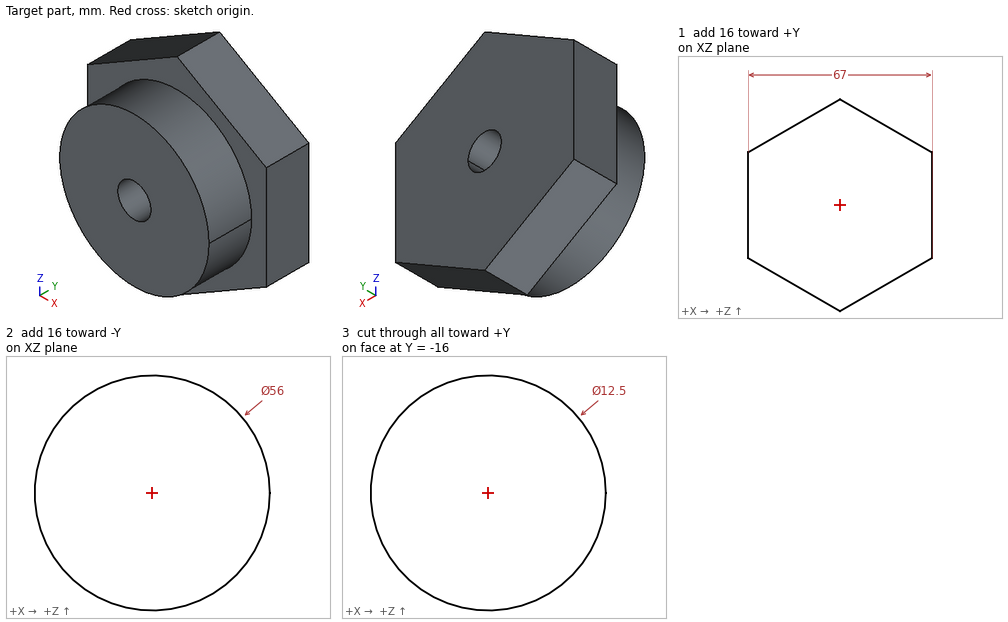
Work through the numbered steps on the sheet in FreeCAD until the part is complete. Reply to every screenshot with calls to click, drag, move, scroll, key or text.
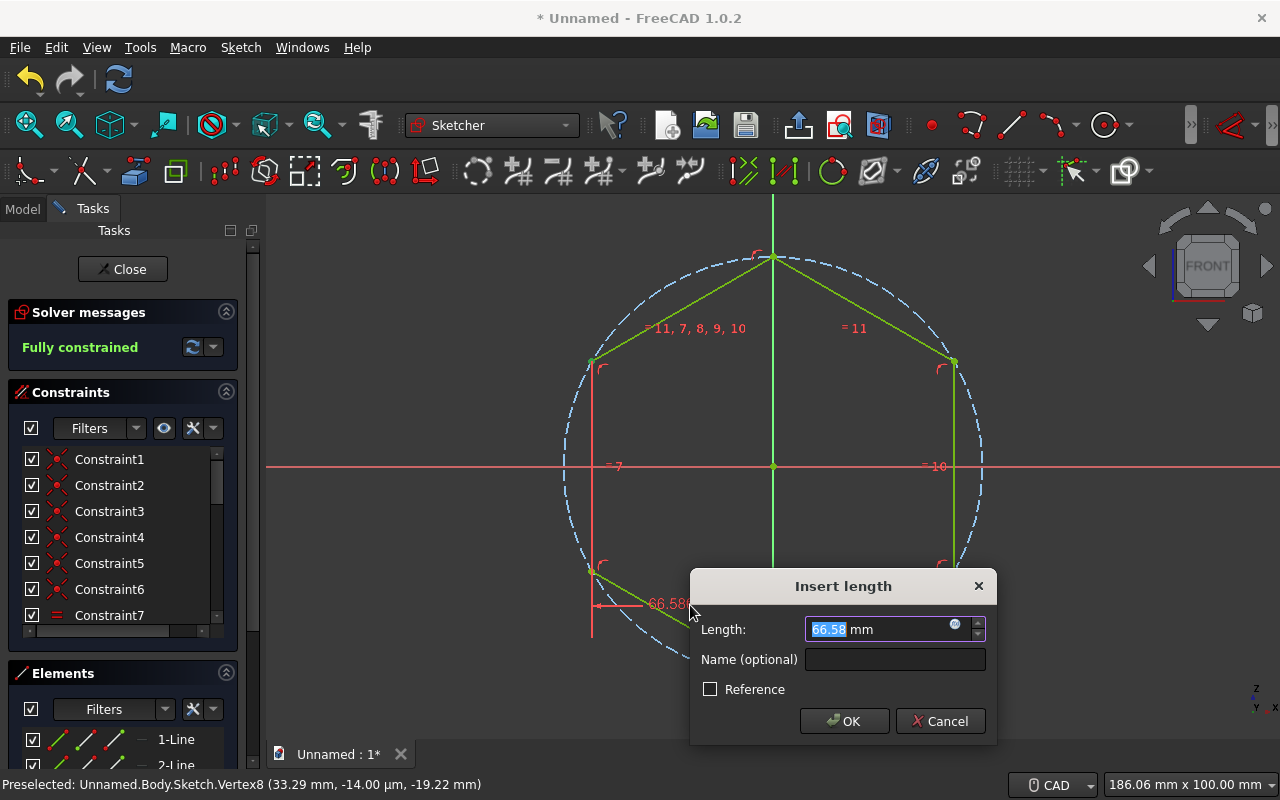
text(67)
key(Return)
key(Escape)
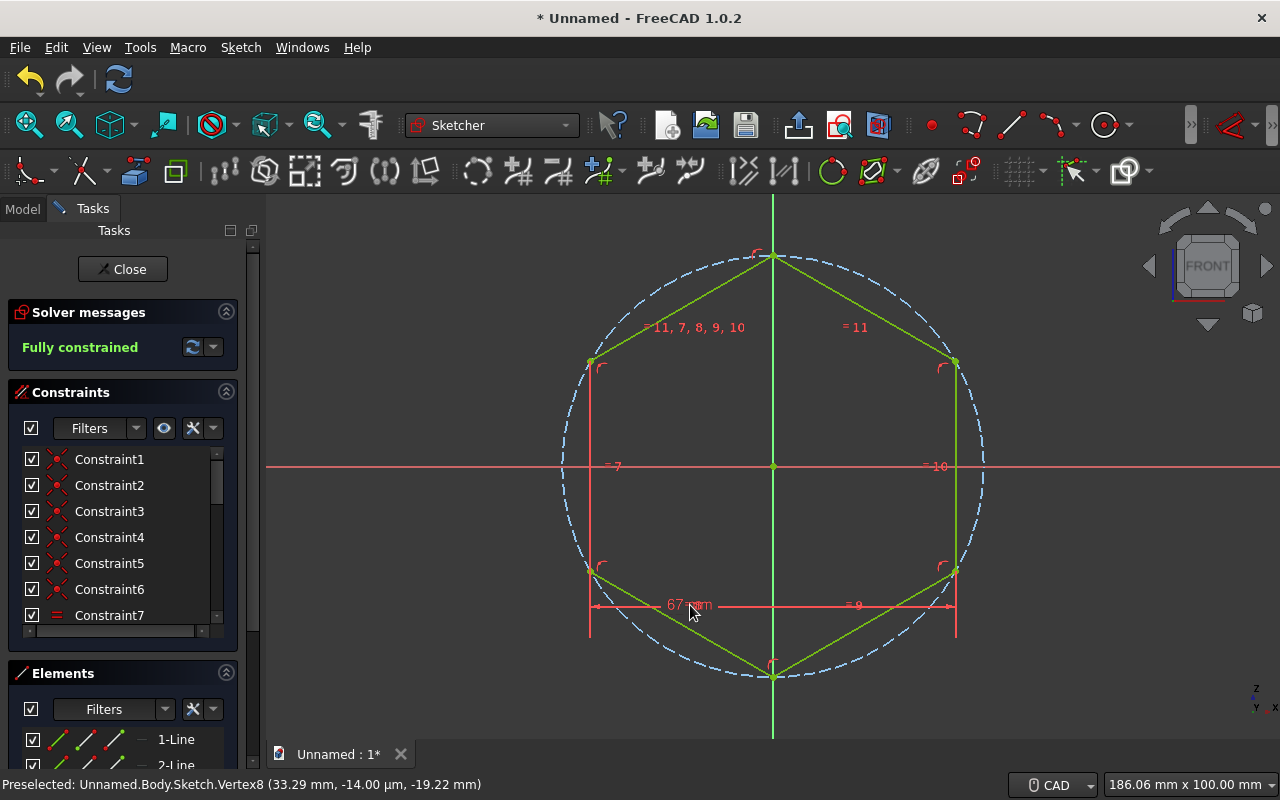
click(123, 269)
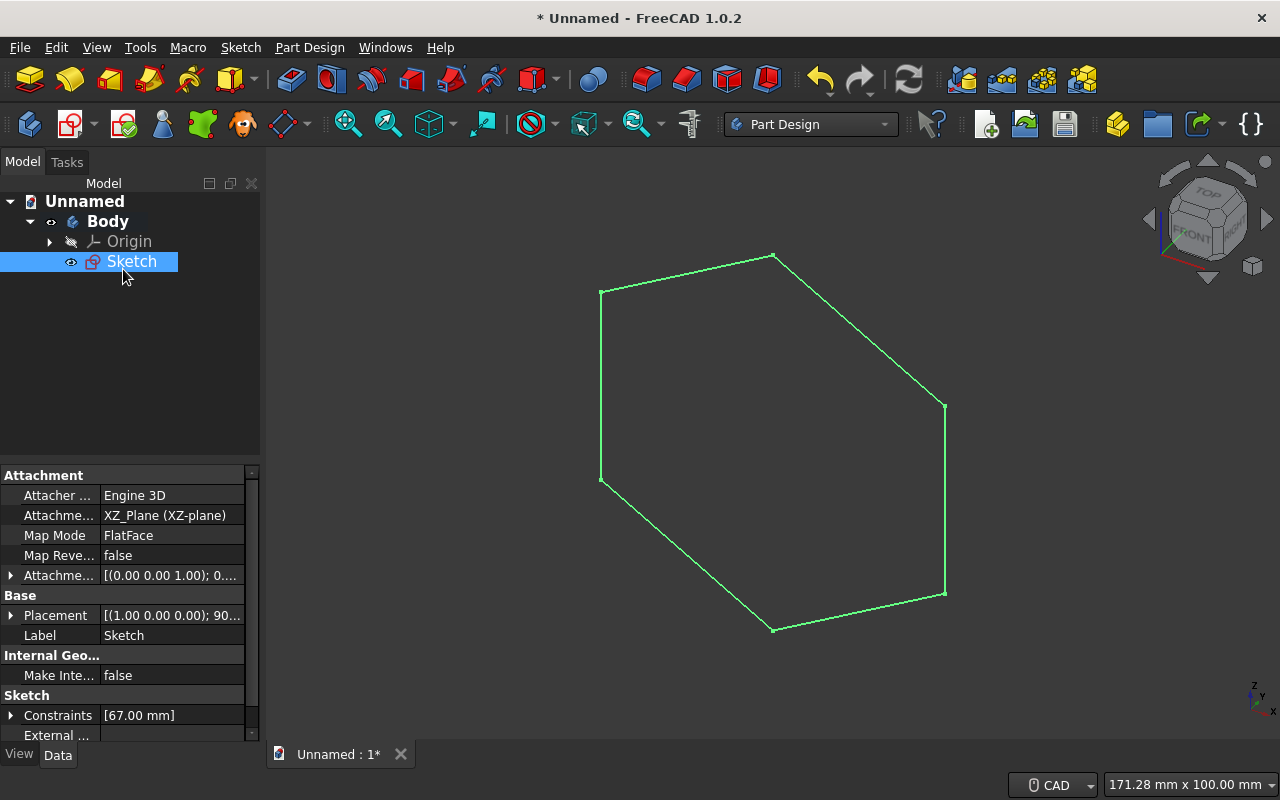
click(30, 80)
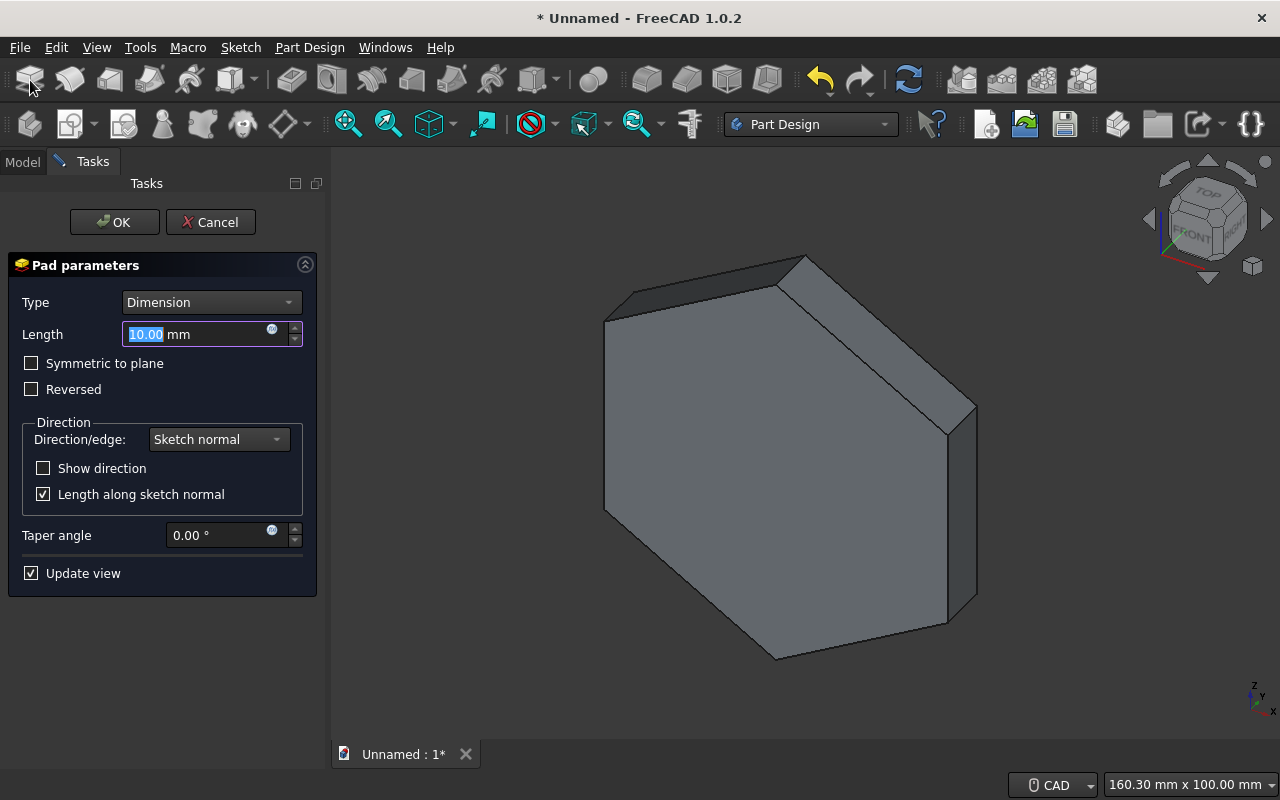
text(16)
key(Tab)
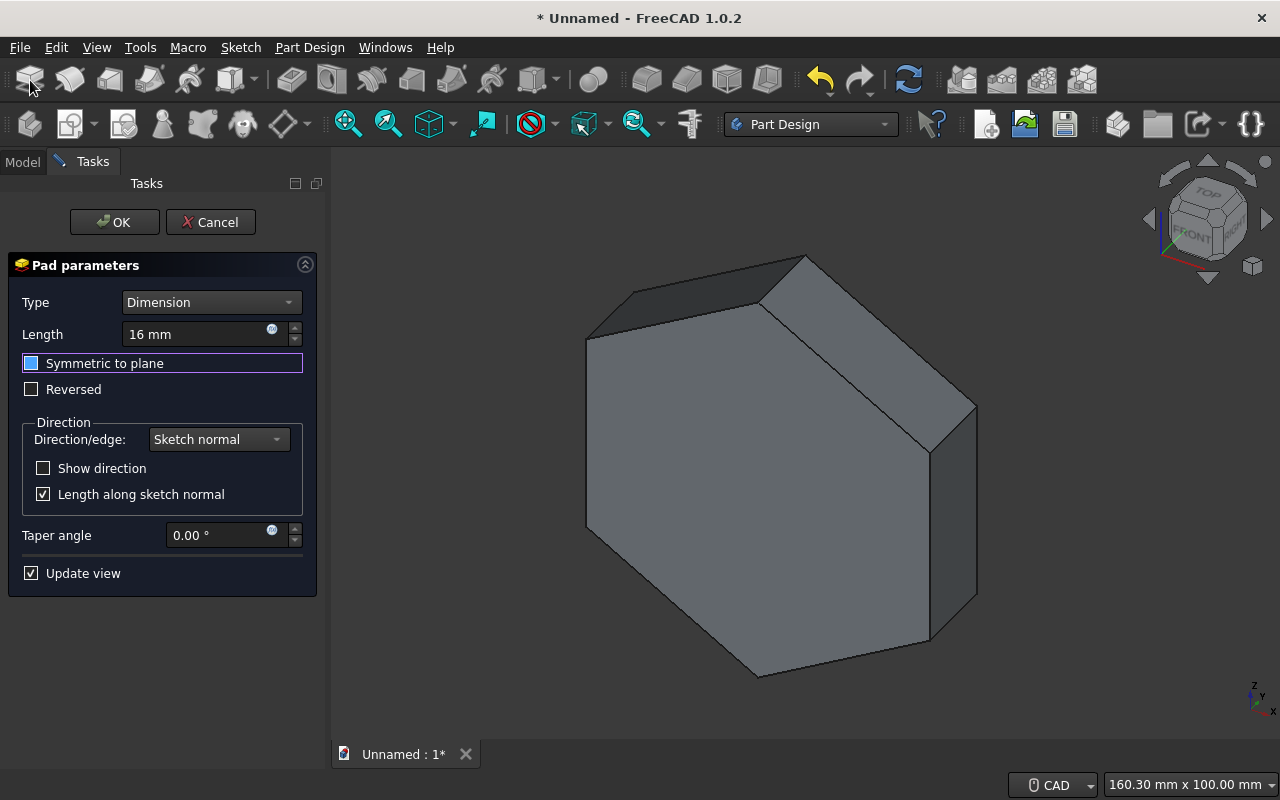
click(30, 389)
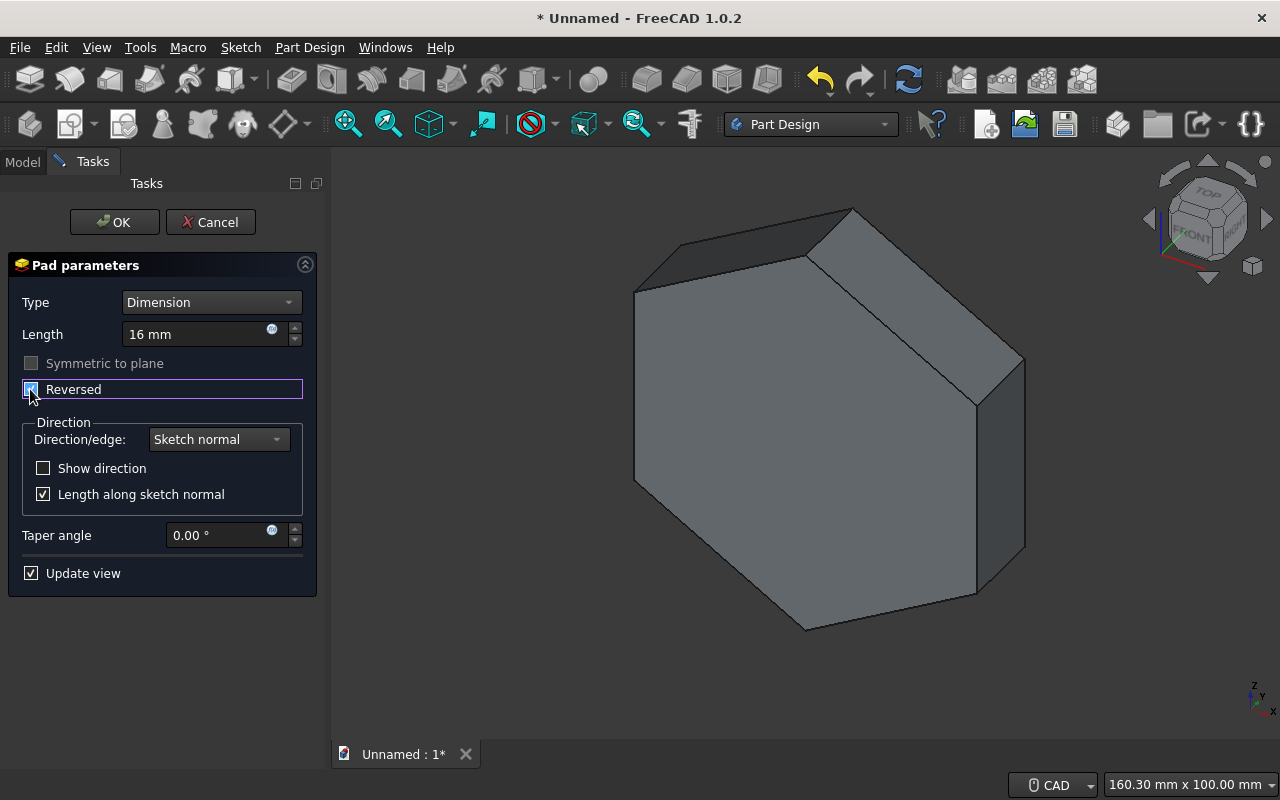
click(115, 222)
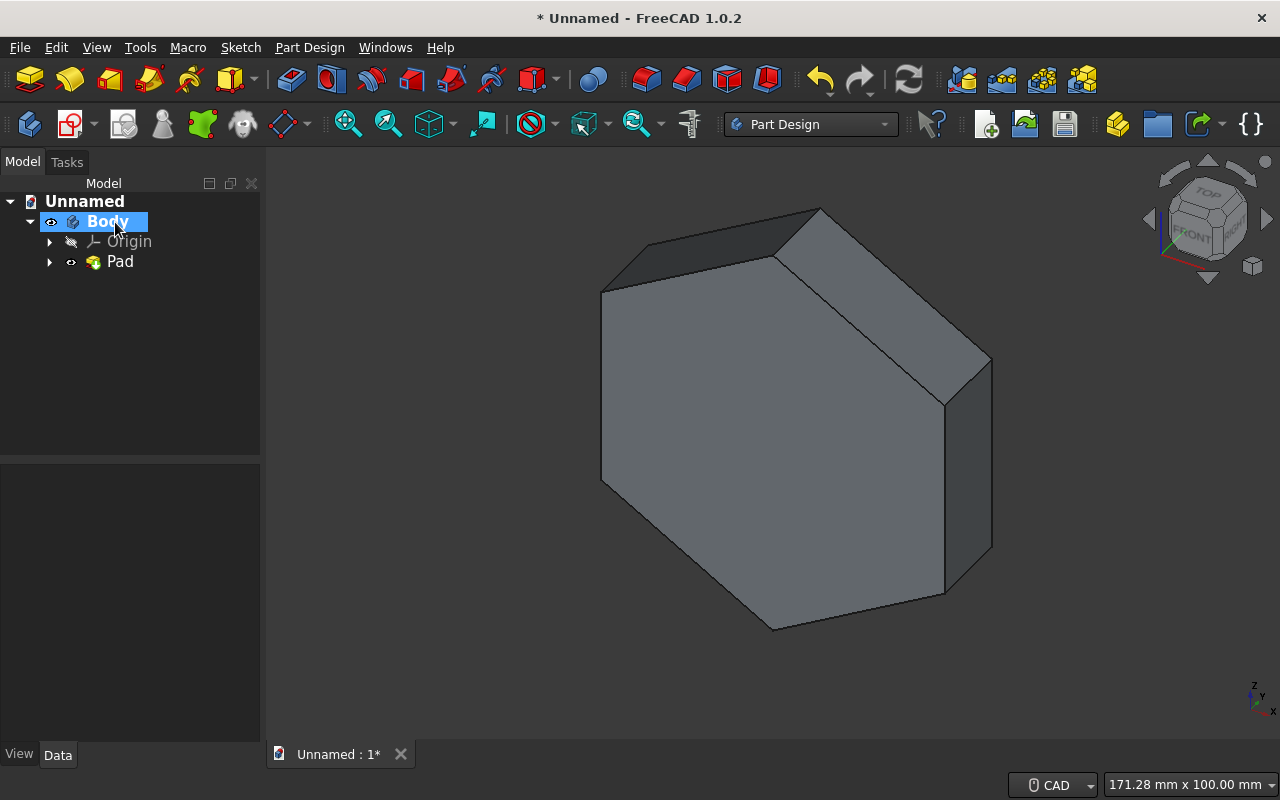
click(70, 124)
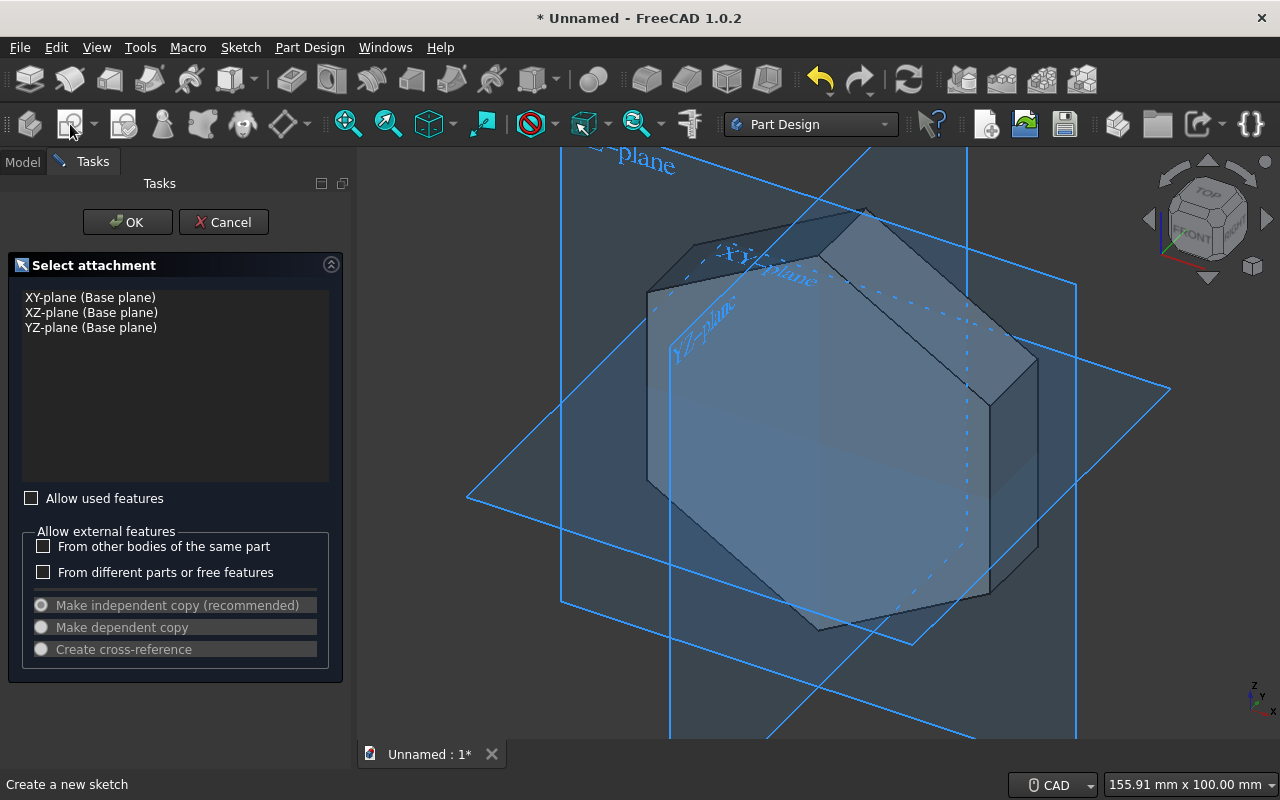
click(82, 312)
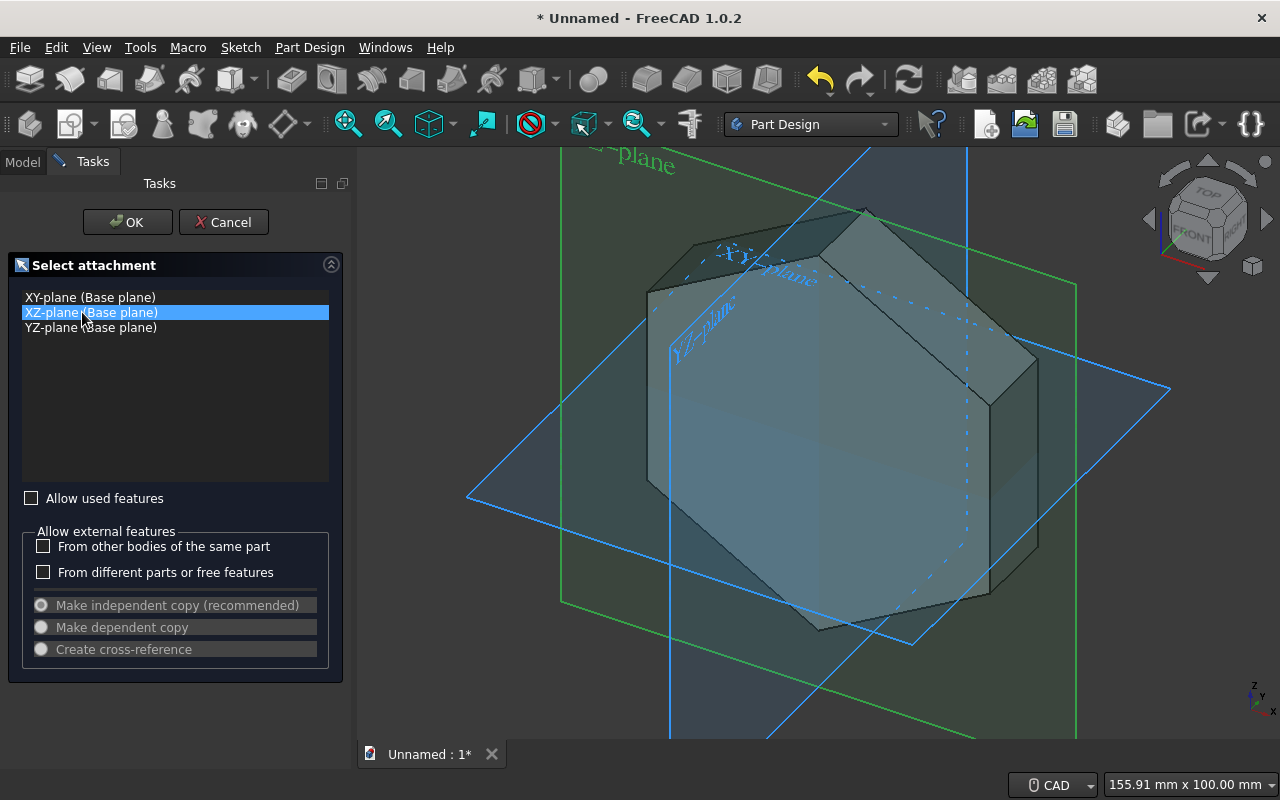
click(128, 222)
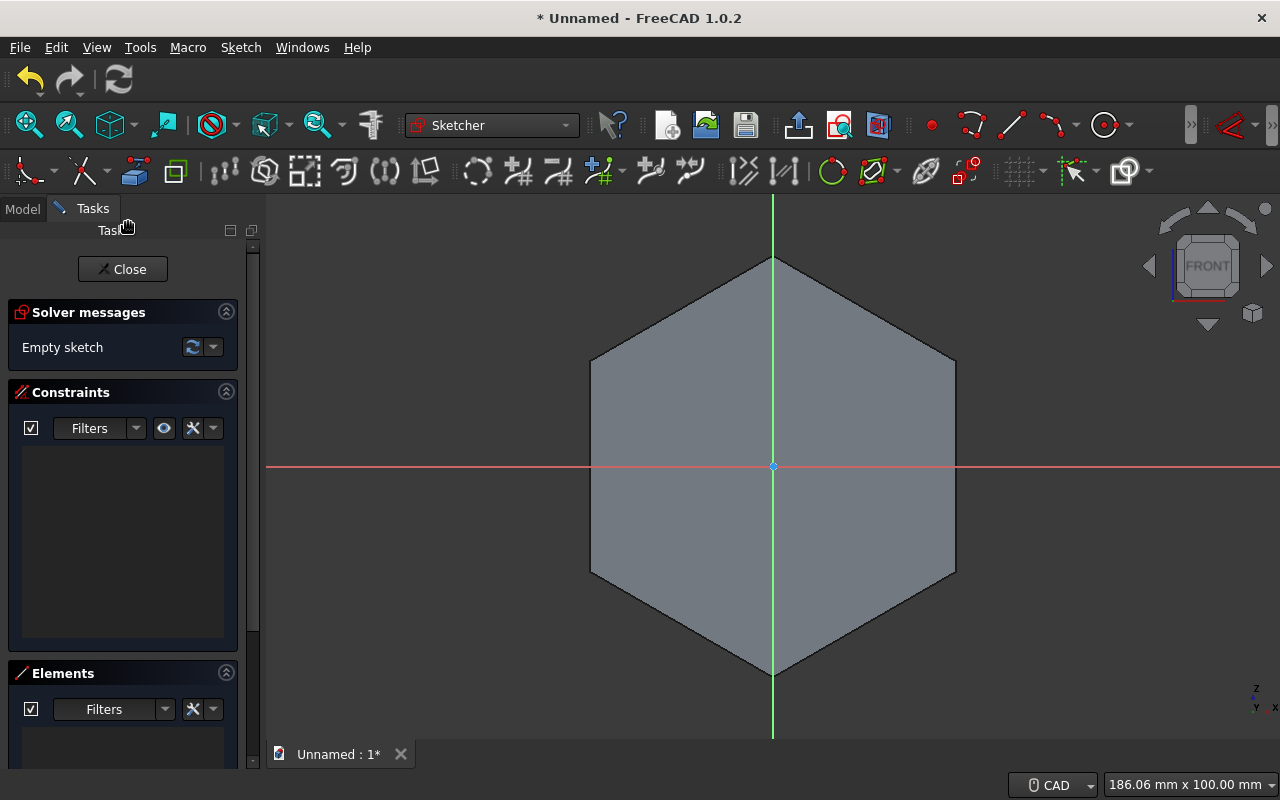
click(1106, 126)